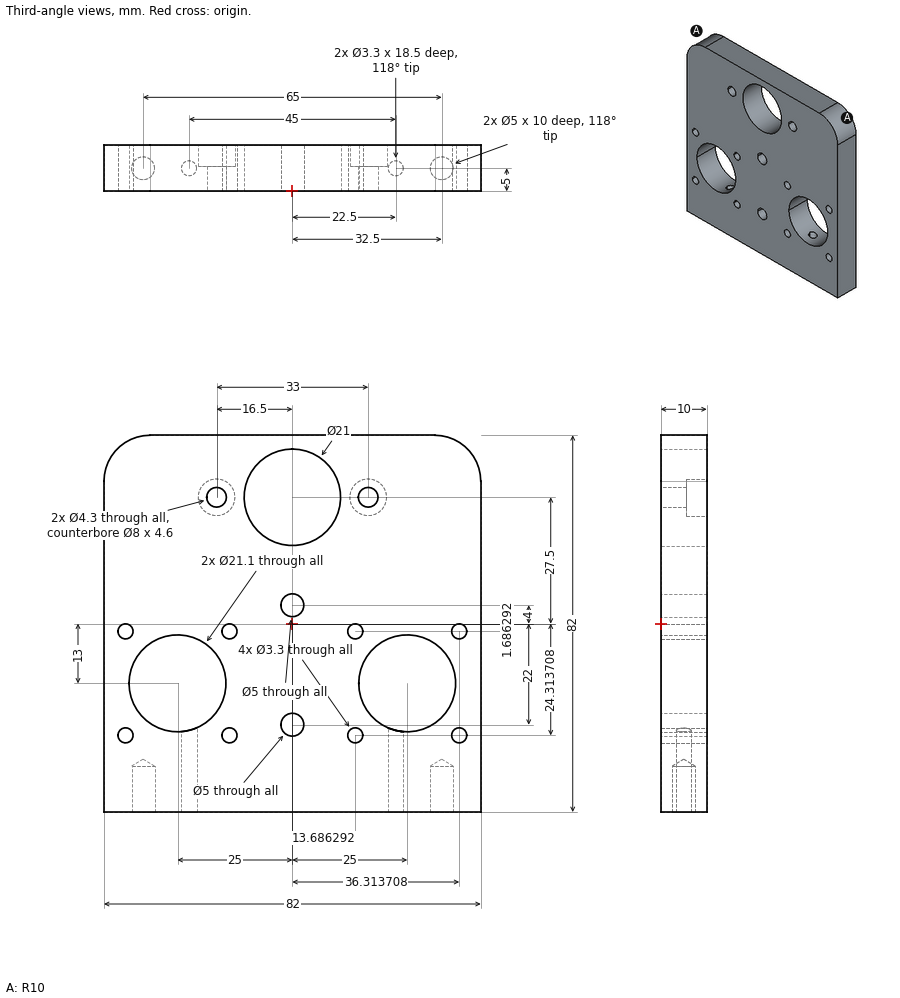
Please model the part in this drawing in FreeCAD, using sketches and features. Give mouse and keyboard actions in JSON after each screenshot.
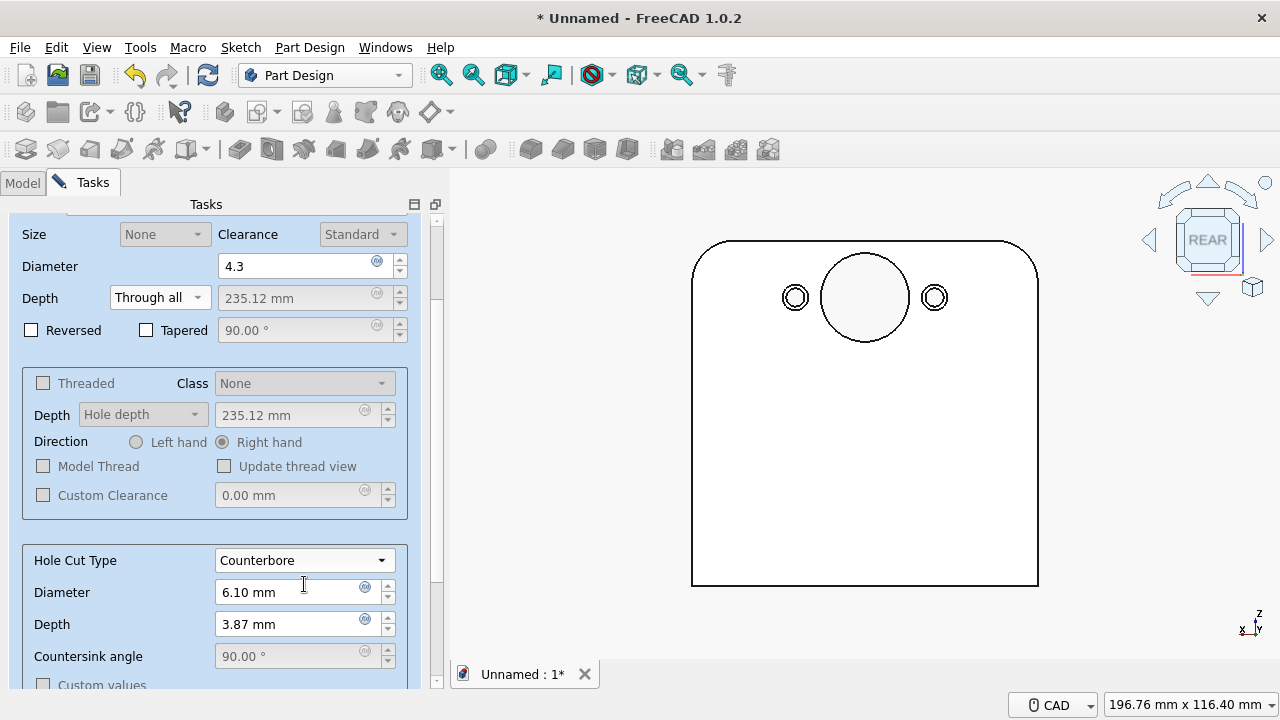
{"action": "triple_click", "coordinate": [298, 592]}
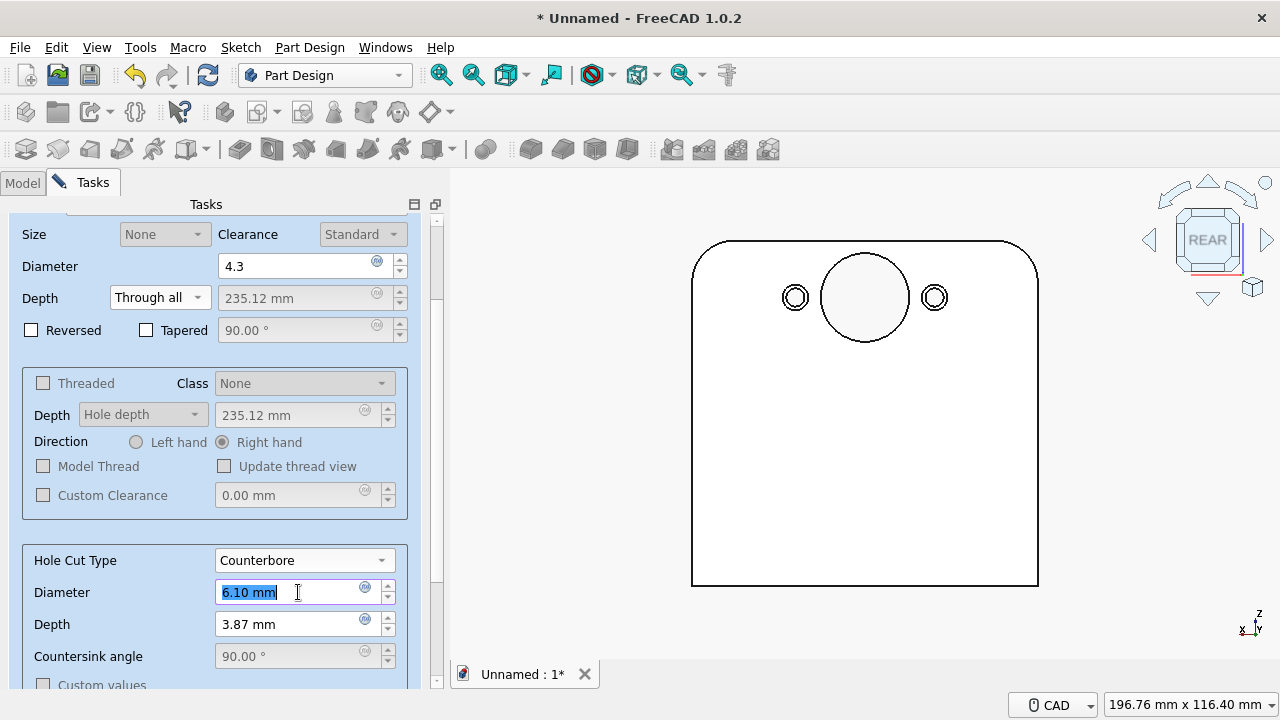
{"action": "type", "text": "8"}
{"action": "key", "text": "Tab"}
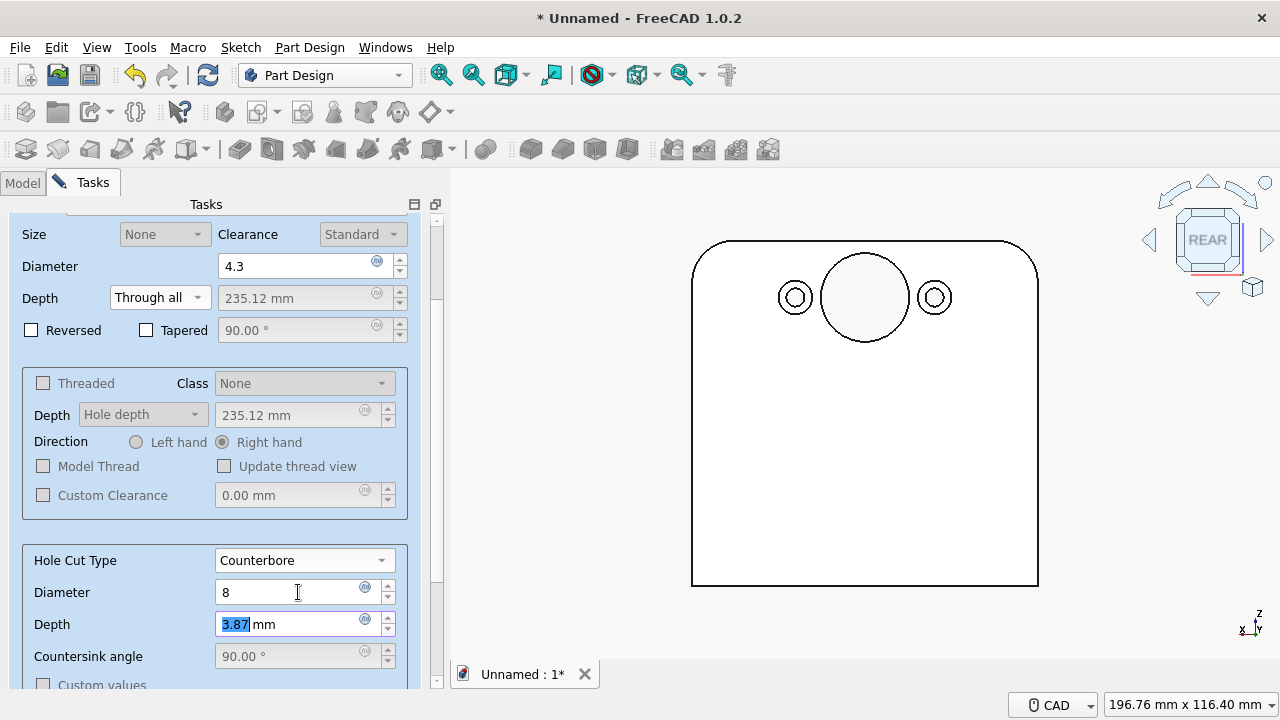
{"action": "type", "text": "4.6"}
{"action": "key", "text": "Tab"}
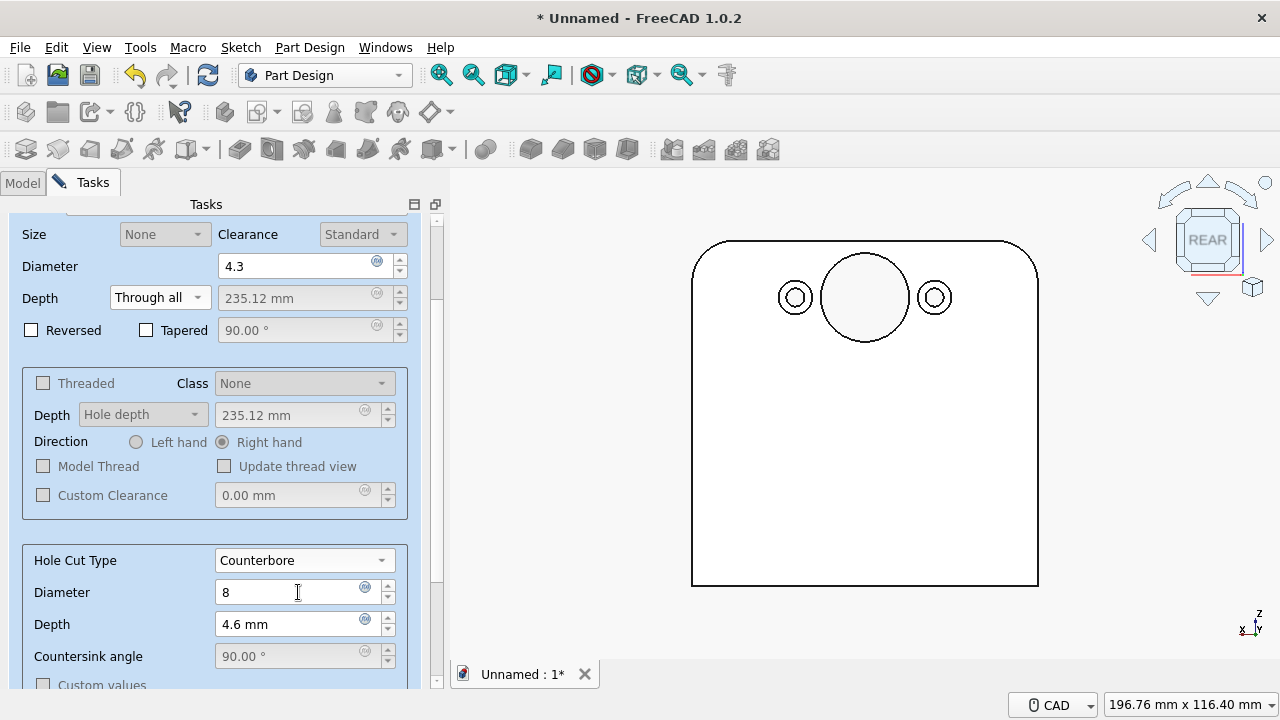
{"action": "scroll", "coordinate": [437, 451], "scroll_direction": "up", "scroll_amount": 3}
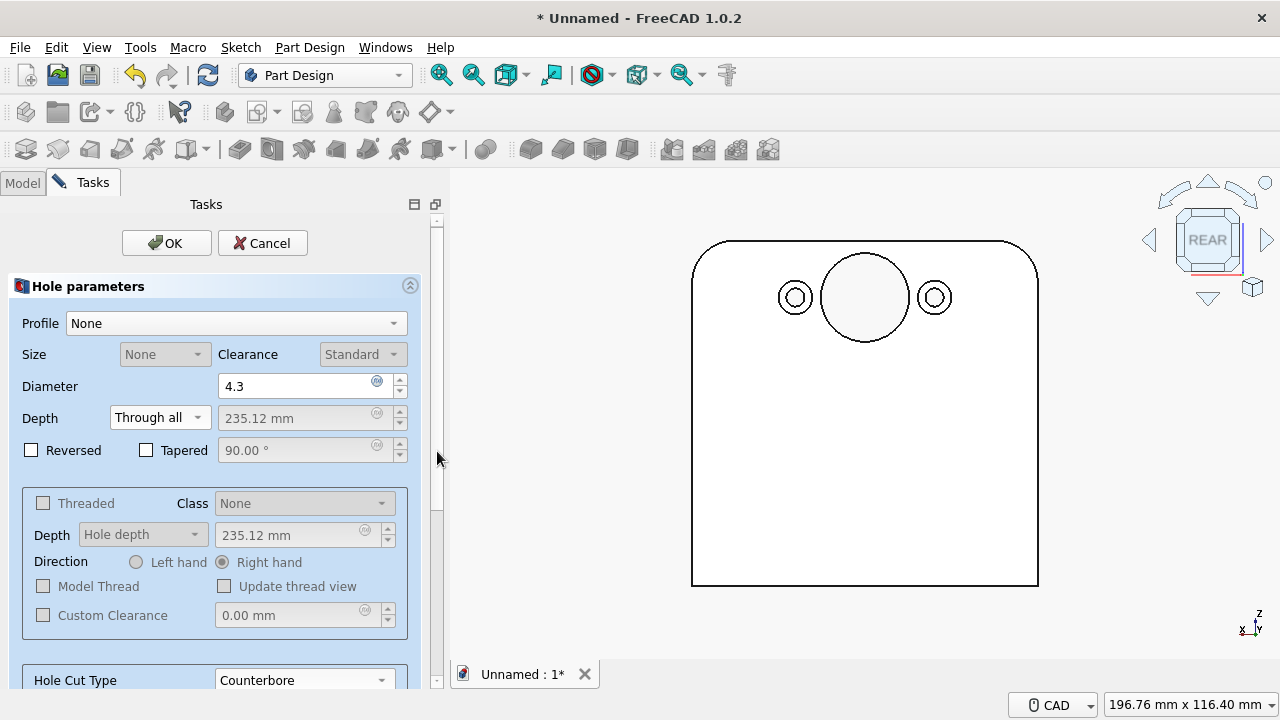
{"action": "left_click", "coordinate": [167, 243]}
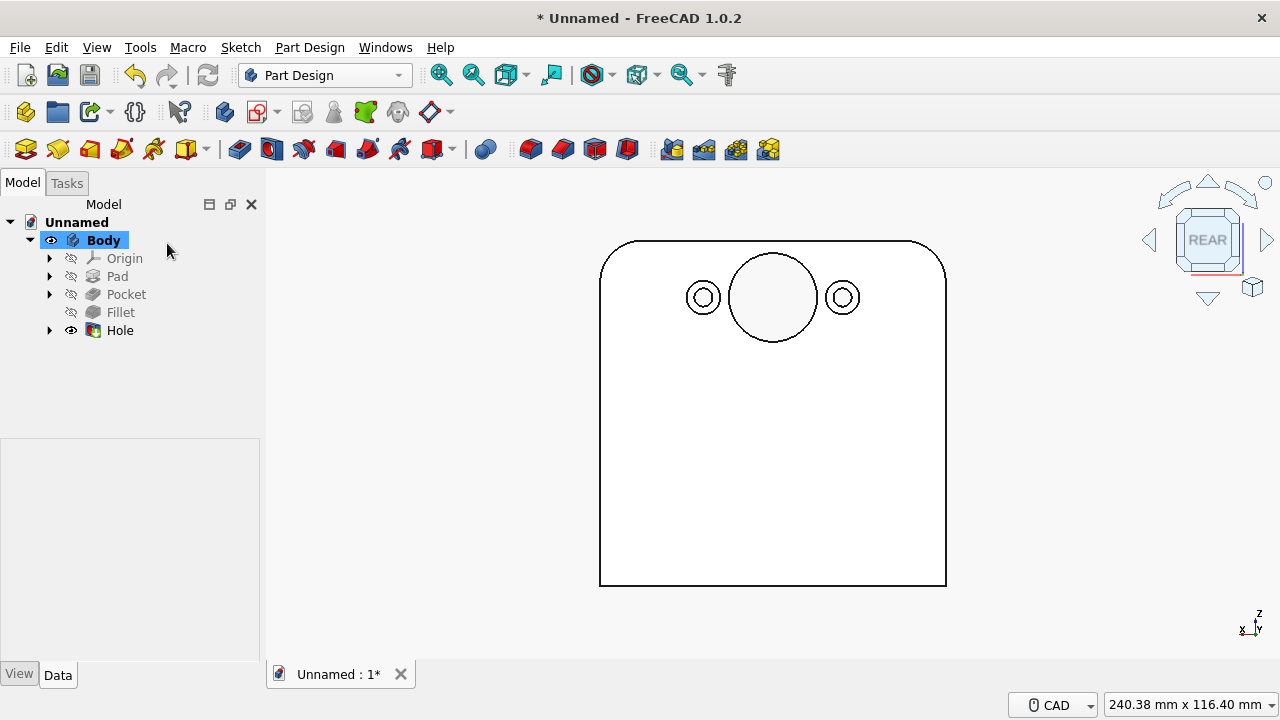
{"action": "key", "text": "5"}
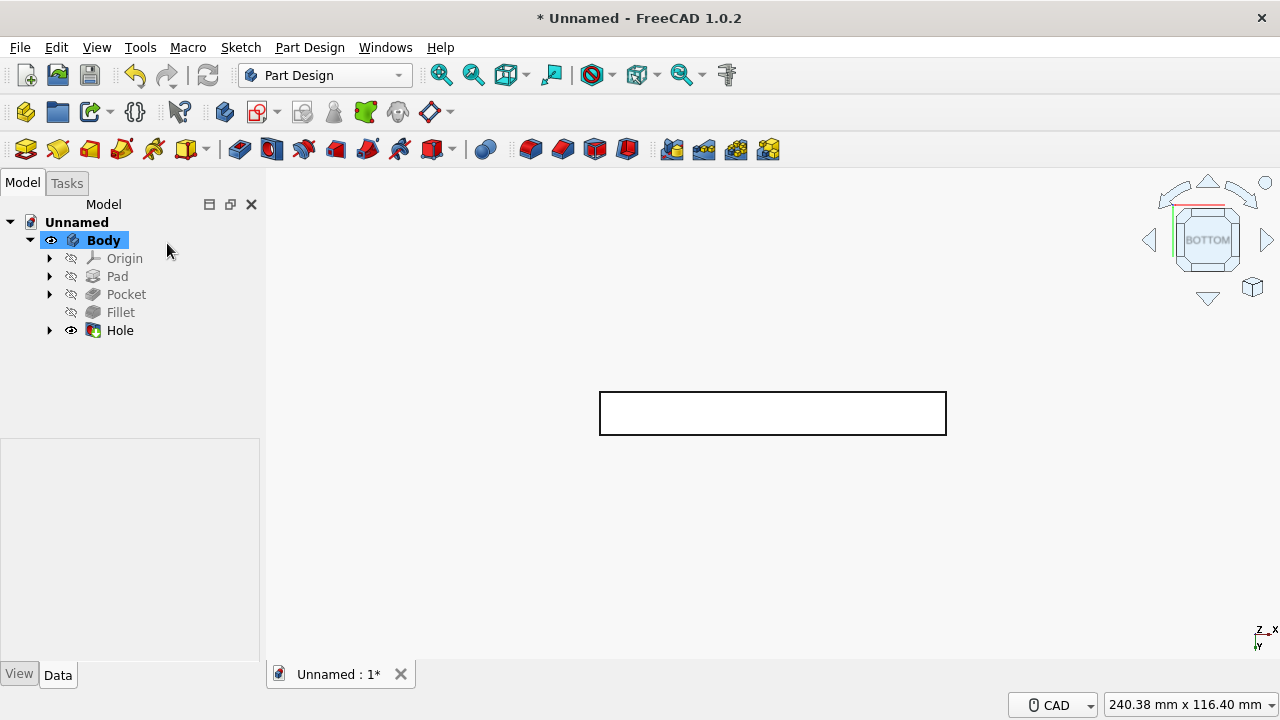
{"action": "left_click", "coordinate": [442, 76]}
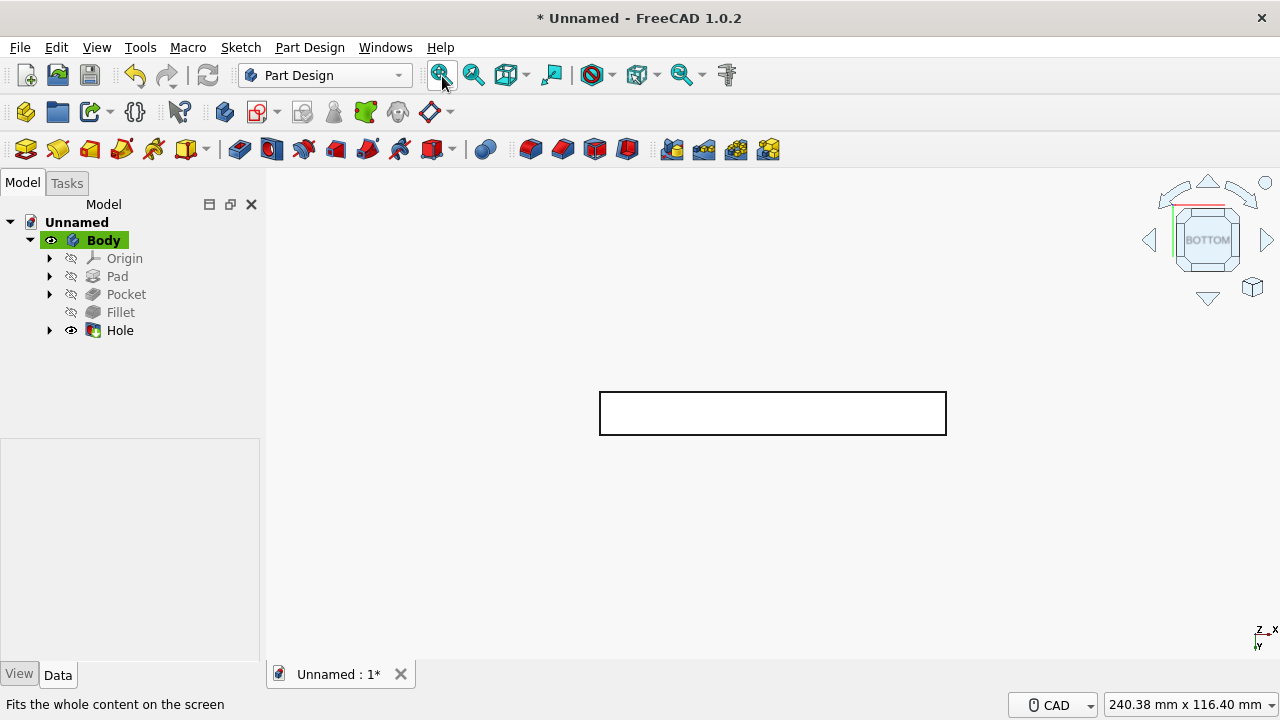
{"action": "left_click", "coordinate": [921, 412]}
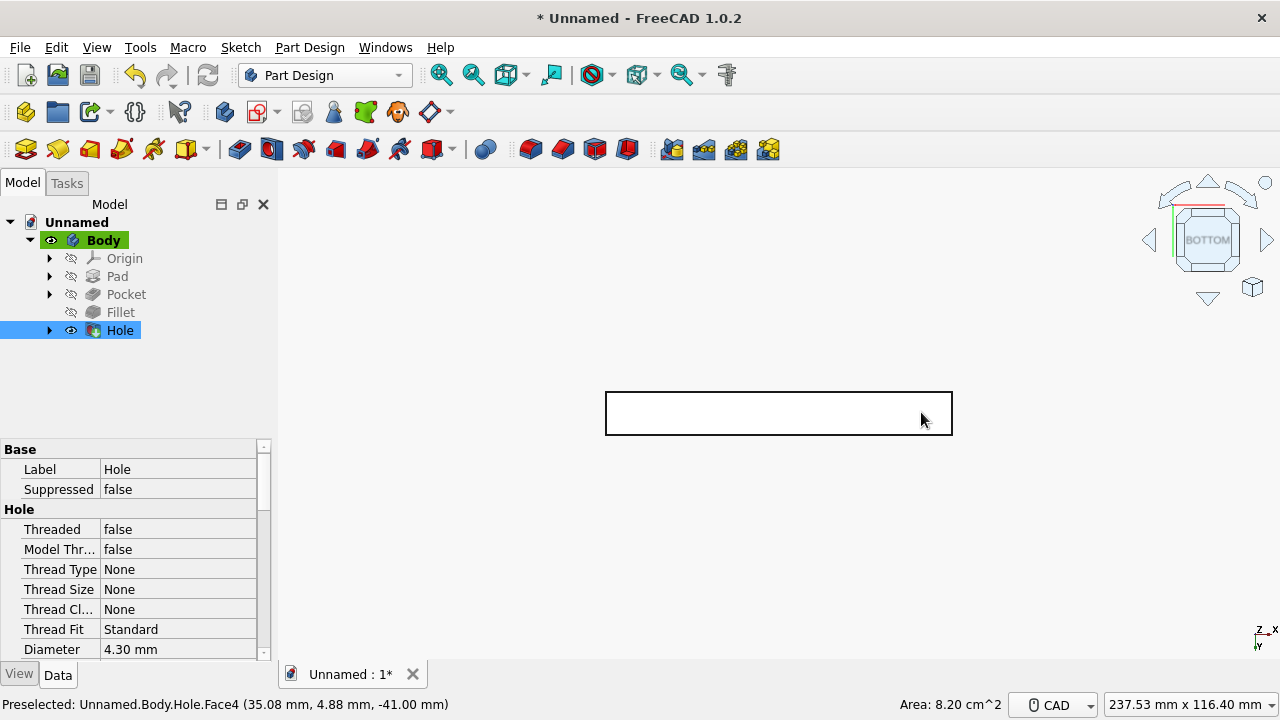
{"action": "left_click", "coordinate": [258, 112]}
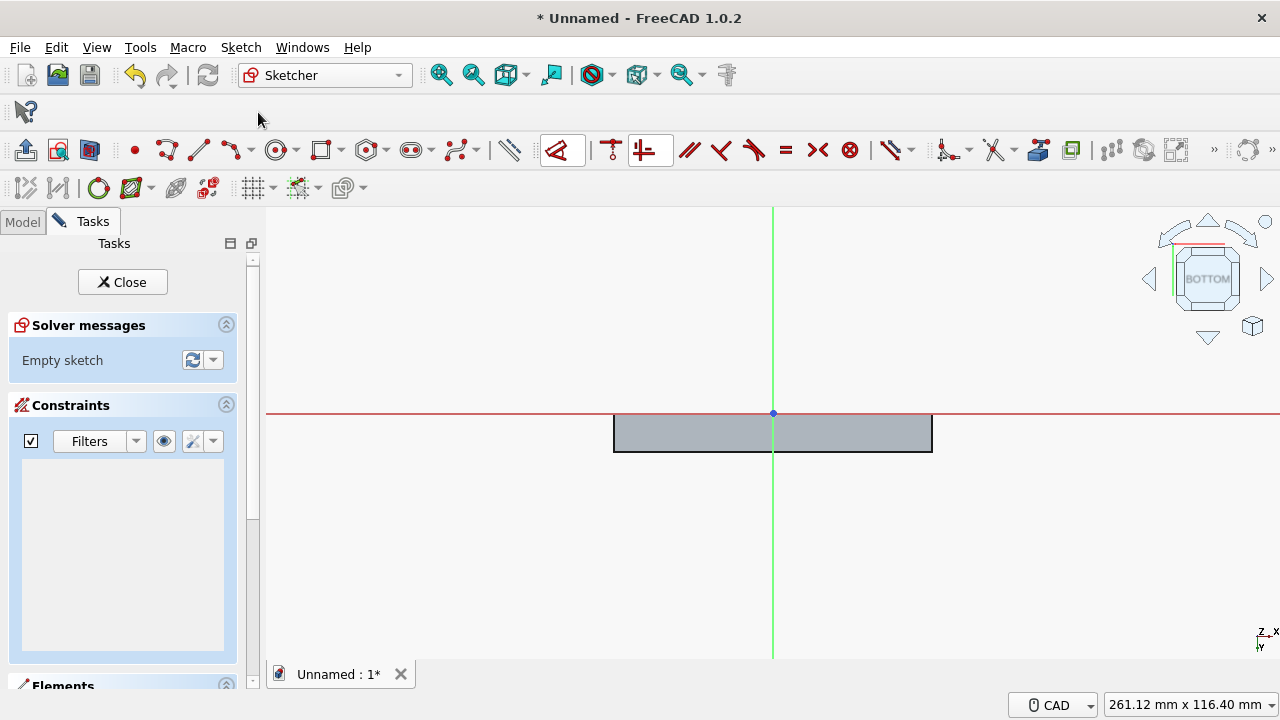
{"action": "scroll", "coordinate": [803, 424], "scroll_direction": "up", "scroll_amount": 6}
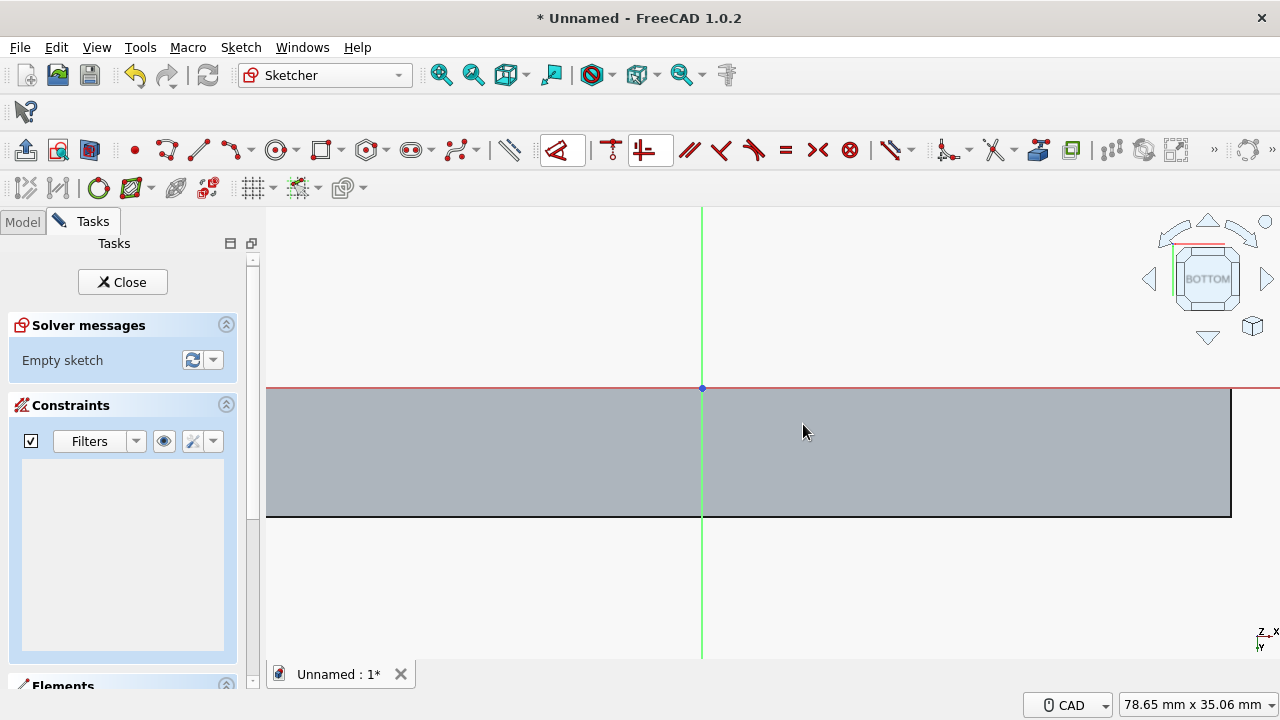
{"action": "left_click", "coordinate": [276, 150]}